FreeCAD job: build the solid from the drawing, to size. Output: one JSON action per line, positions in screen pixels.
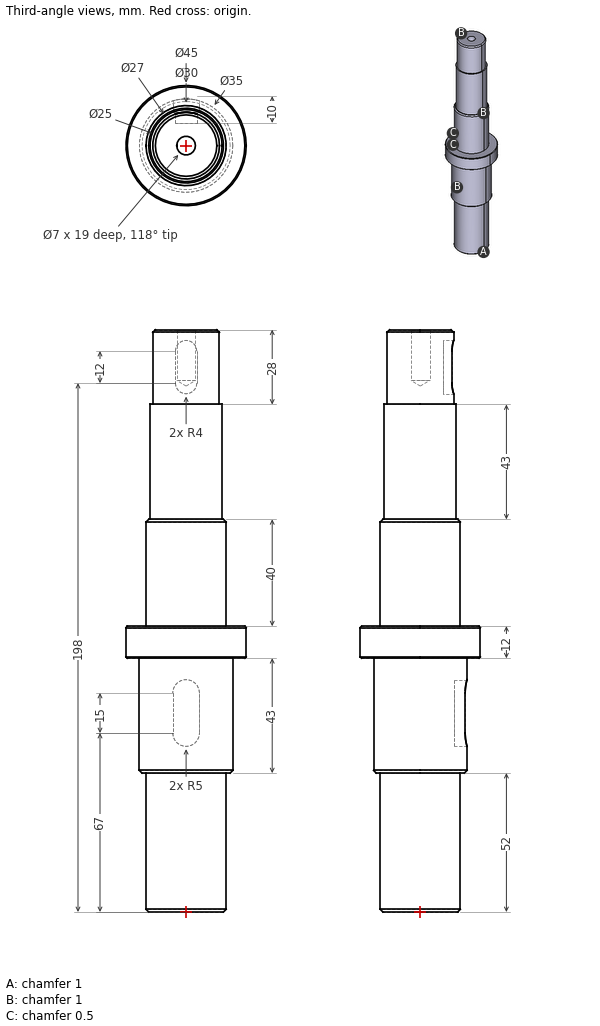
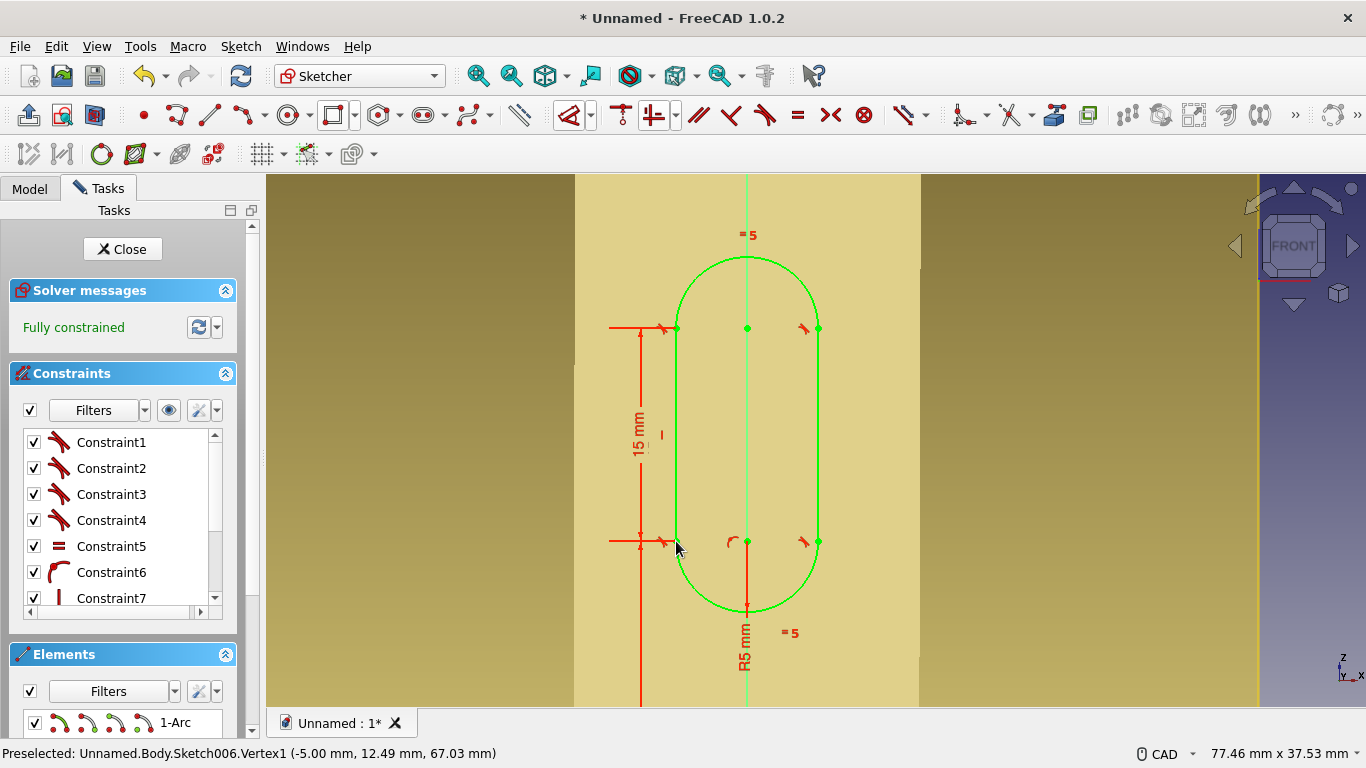
{"action": "left_click", "coordinate": [123, 249]}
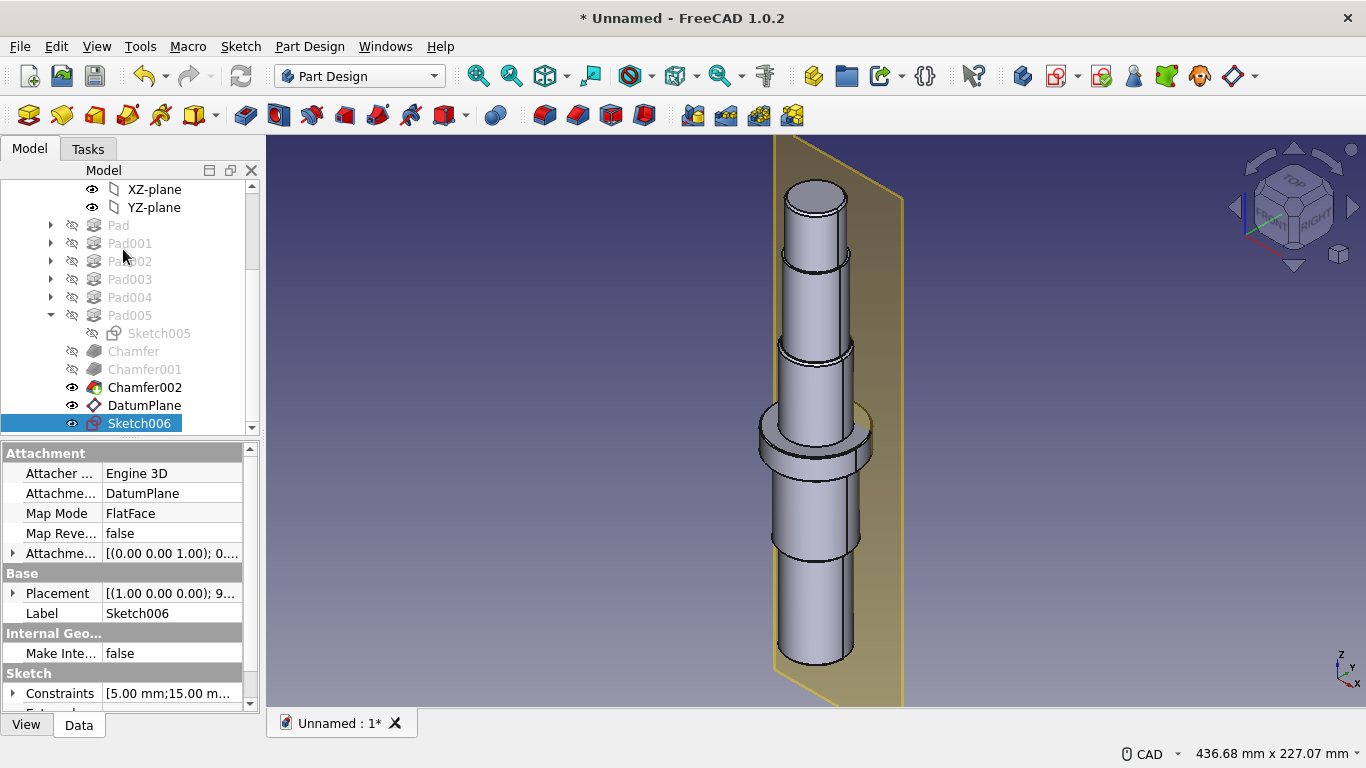
{"action": "left_click", "coordinate": [246, 116]}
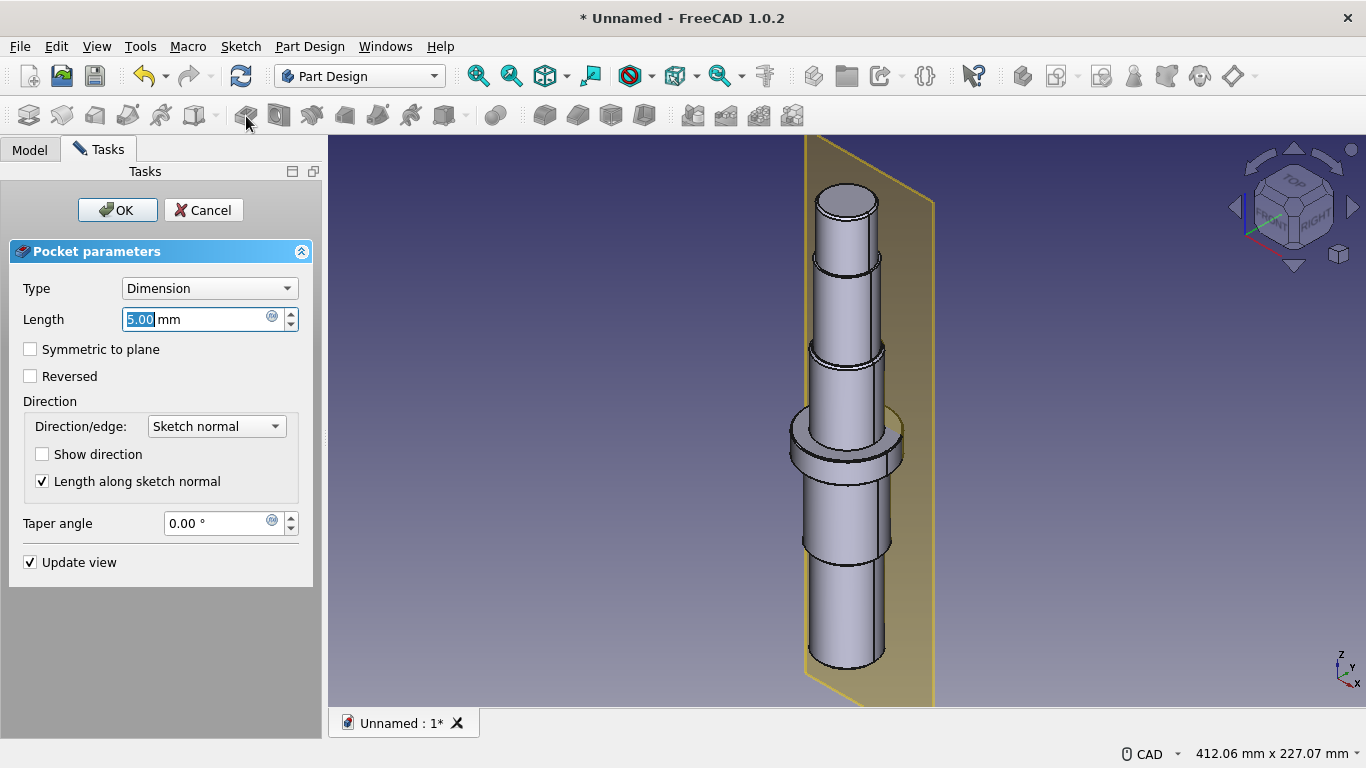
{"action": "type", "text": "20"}
{"action": "key", "text": "Tab"}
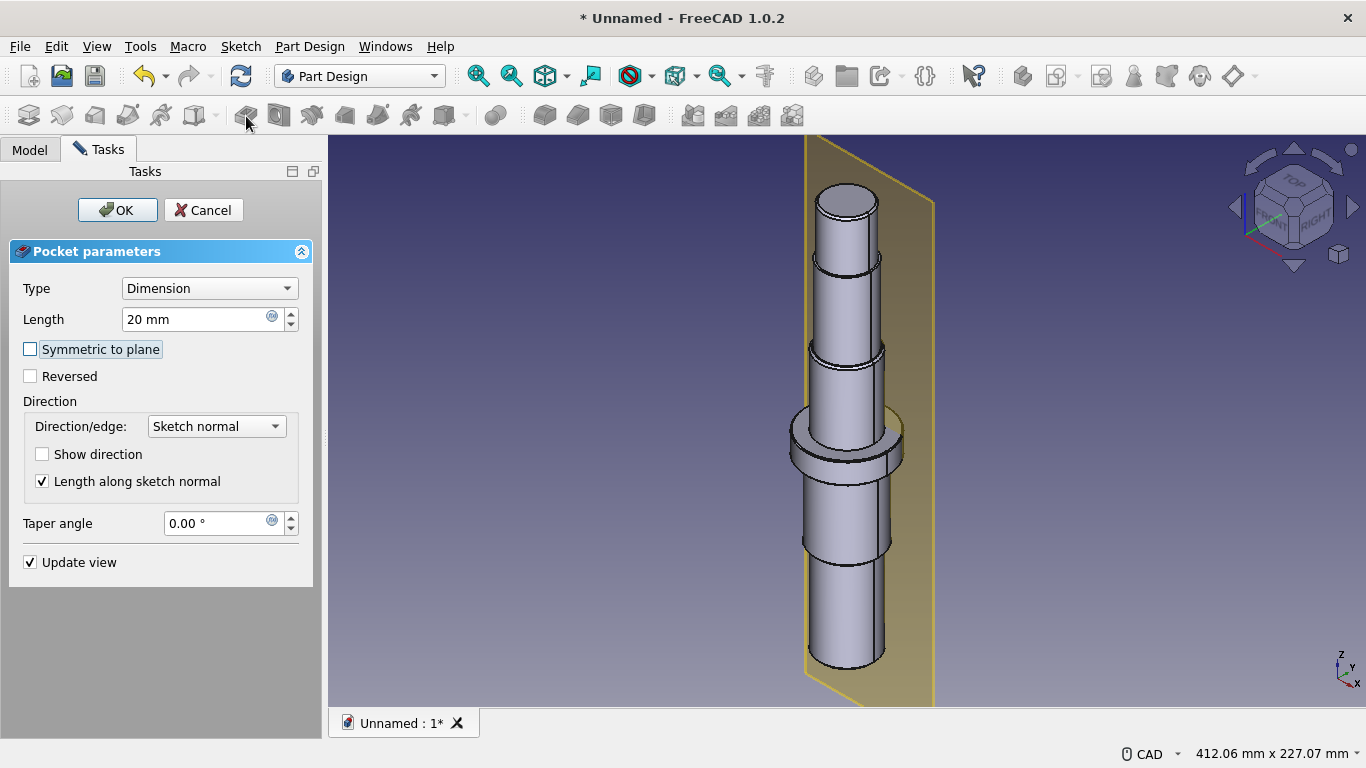
{"action": "left_click", "coordinate": [118, 210]}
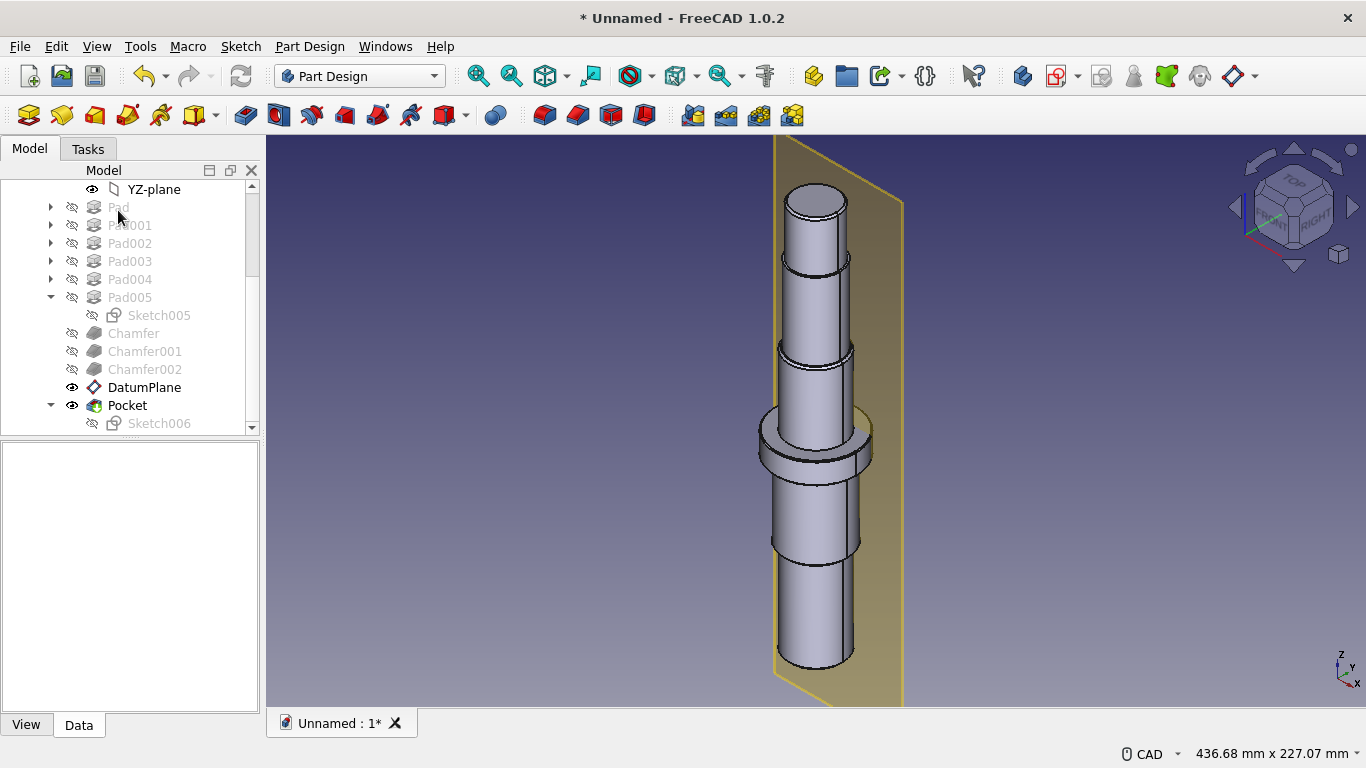
{"action": "left_click", "coordinate": [117, 387]}
{"action": "key", "text": "space"}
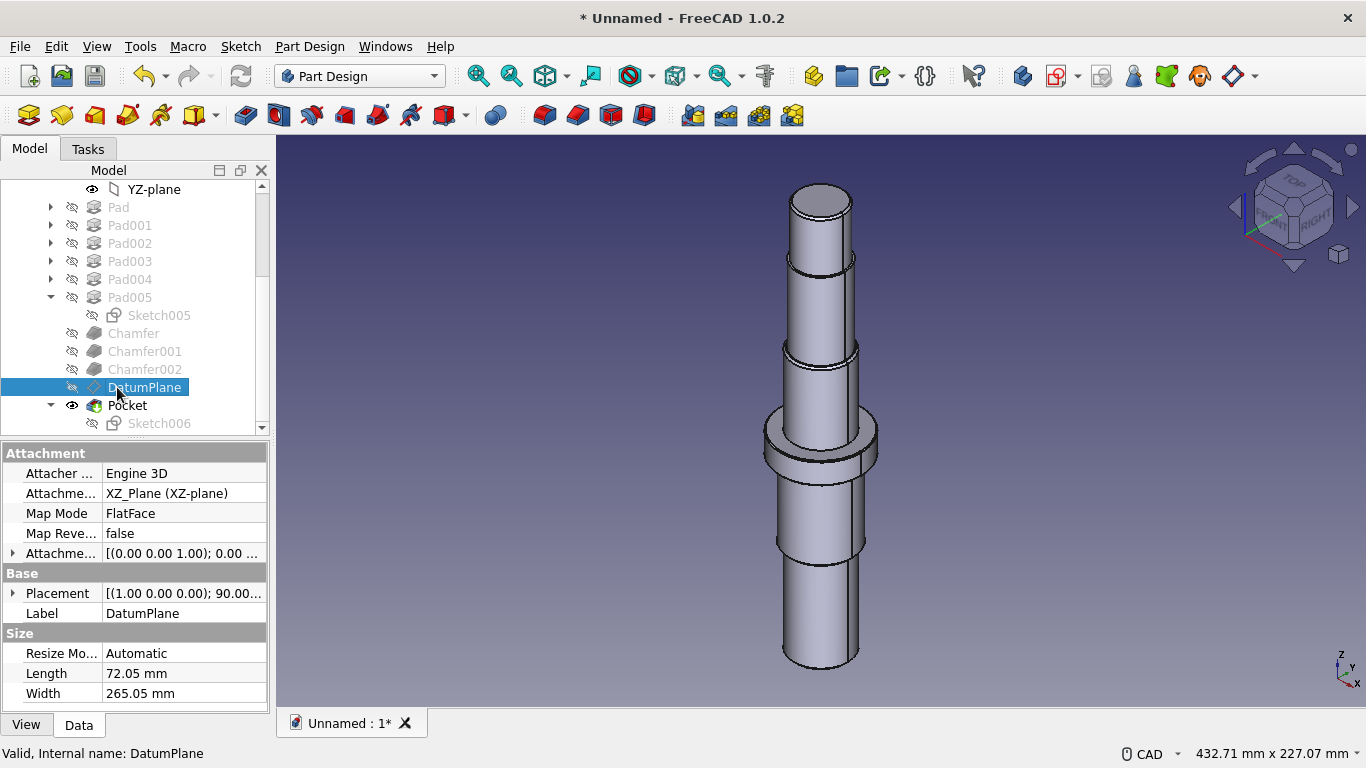
{"action": "scroll", "coordinate": [161, 311], "scroll_direction": "down", "scroll_amount": 3}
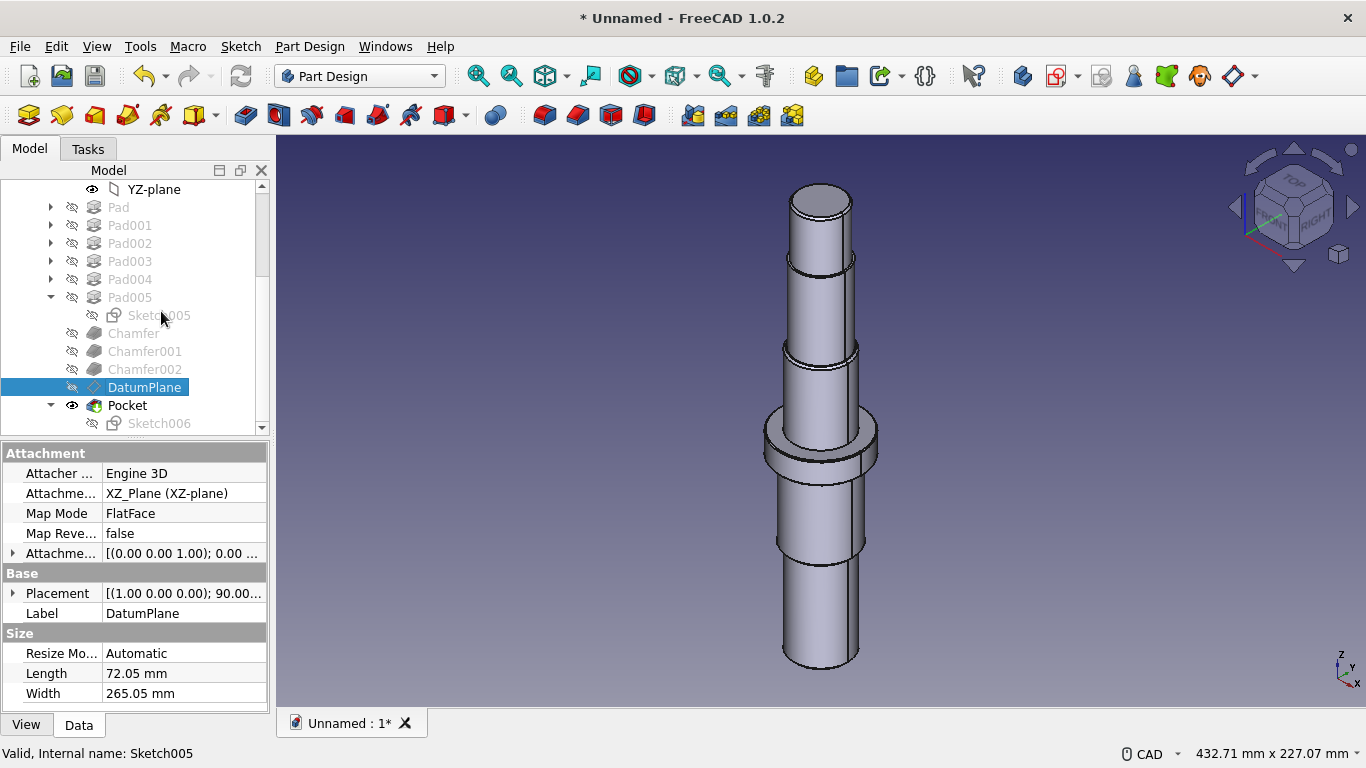
{"action": "scroll", "coordinate": [161, 311], "scroll_direction": "up", "scroll_amount": 15}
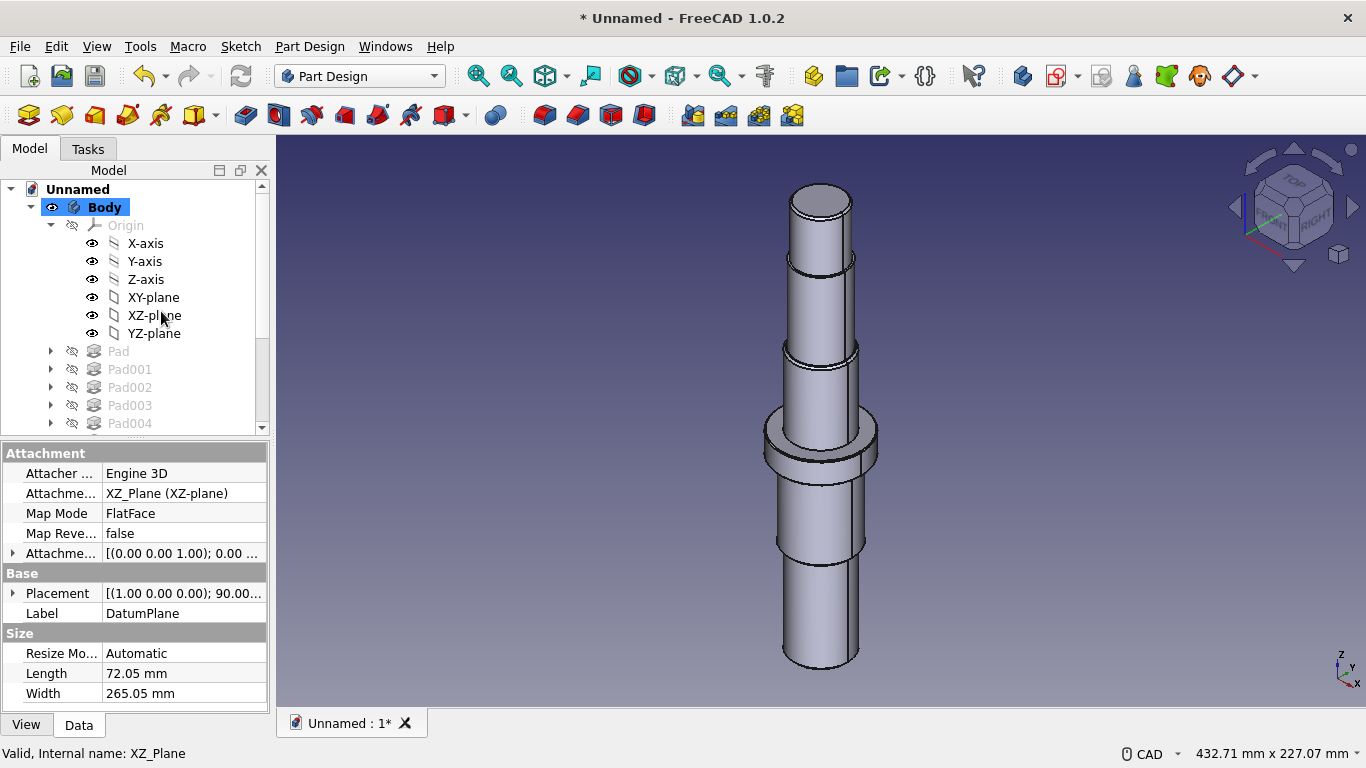
{"action": "left_click", "coordinate": [137, 315]}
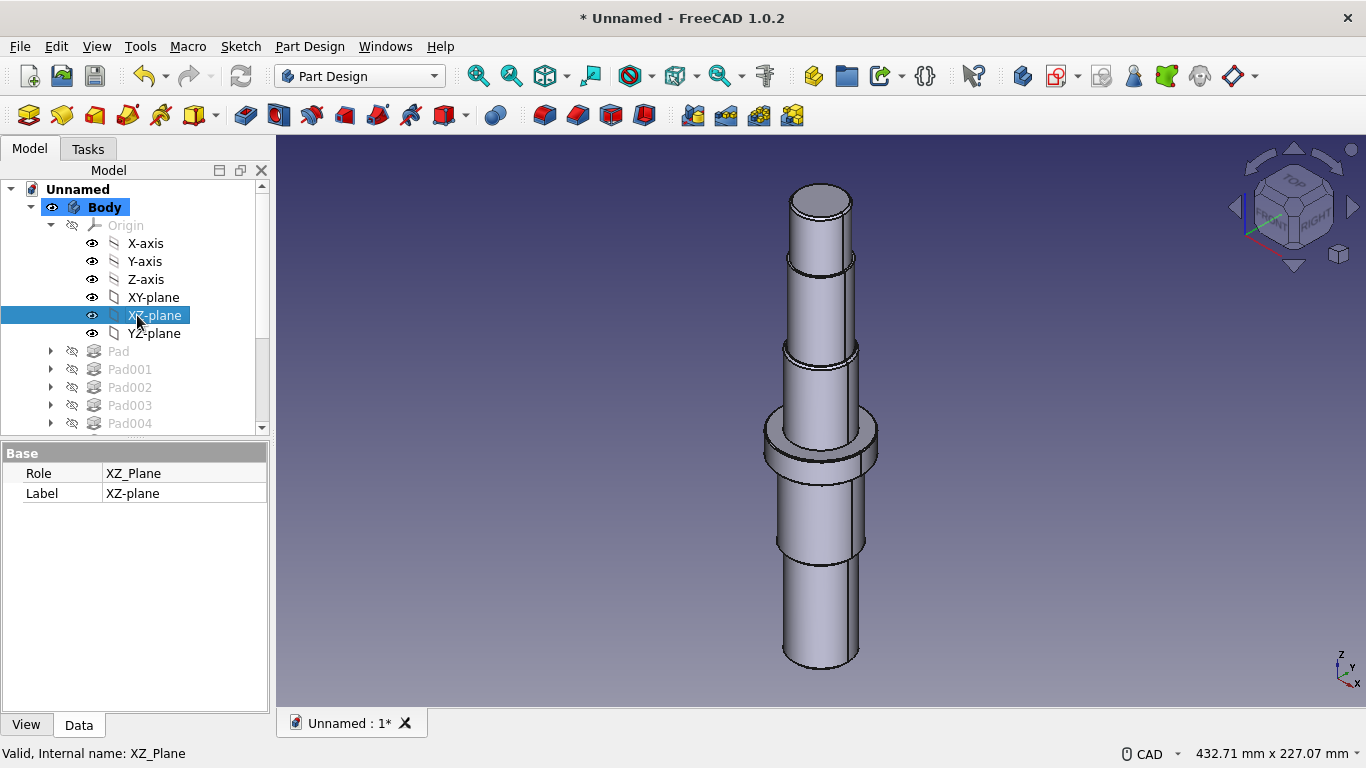
{"action": "left_click", "coordinate": [1232, 76]}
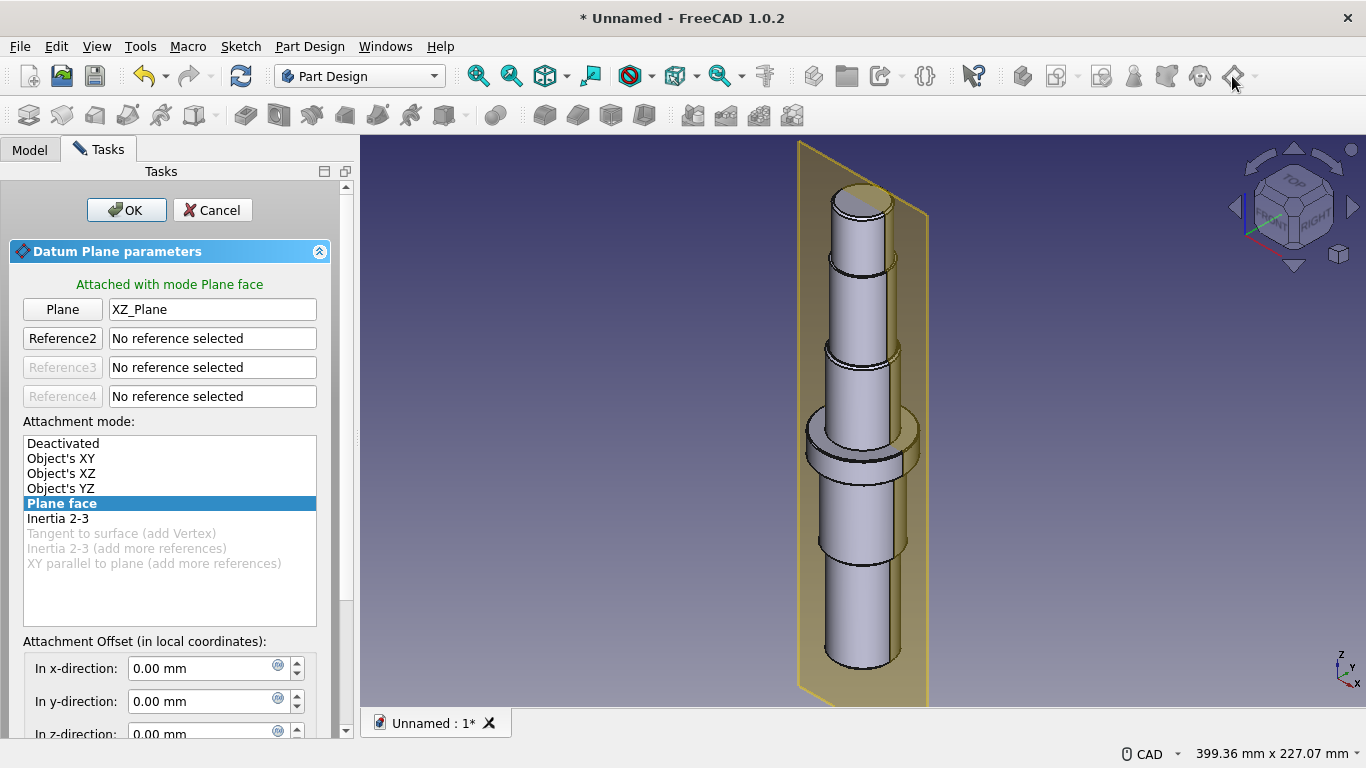
{"action": "scroll", "coordinate": [346, 460], "scroll_direction": "down", "scroll_amount": 2}